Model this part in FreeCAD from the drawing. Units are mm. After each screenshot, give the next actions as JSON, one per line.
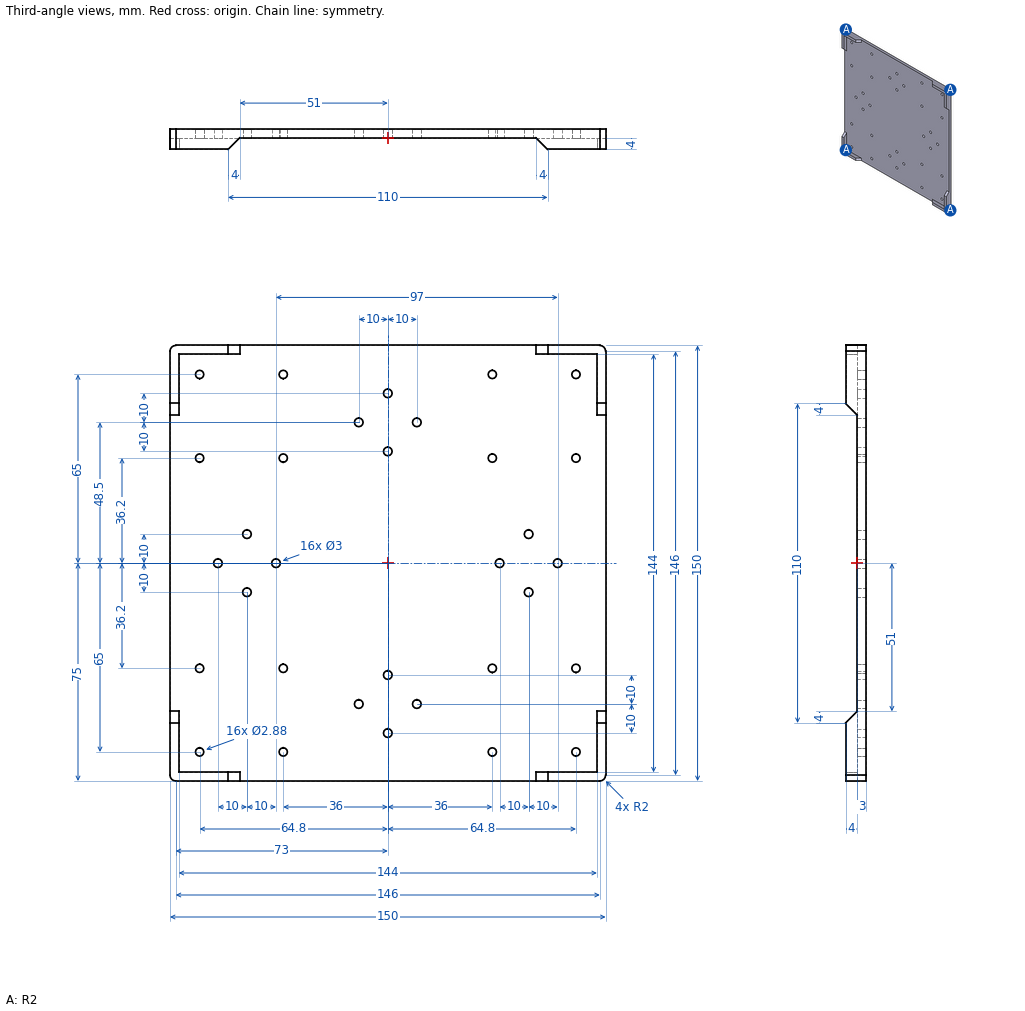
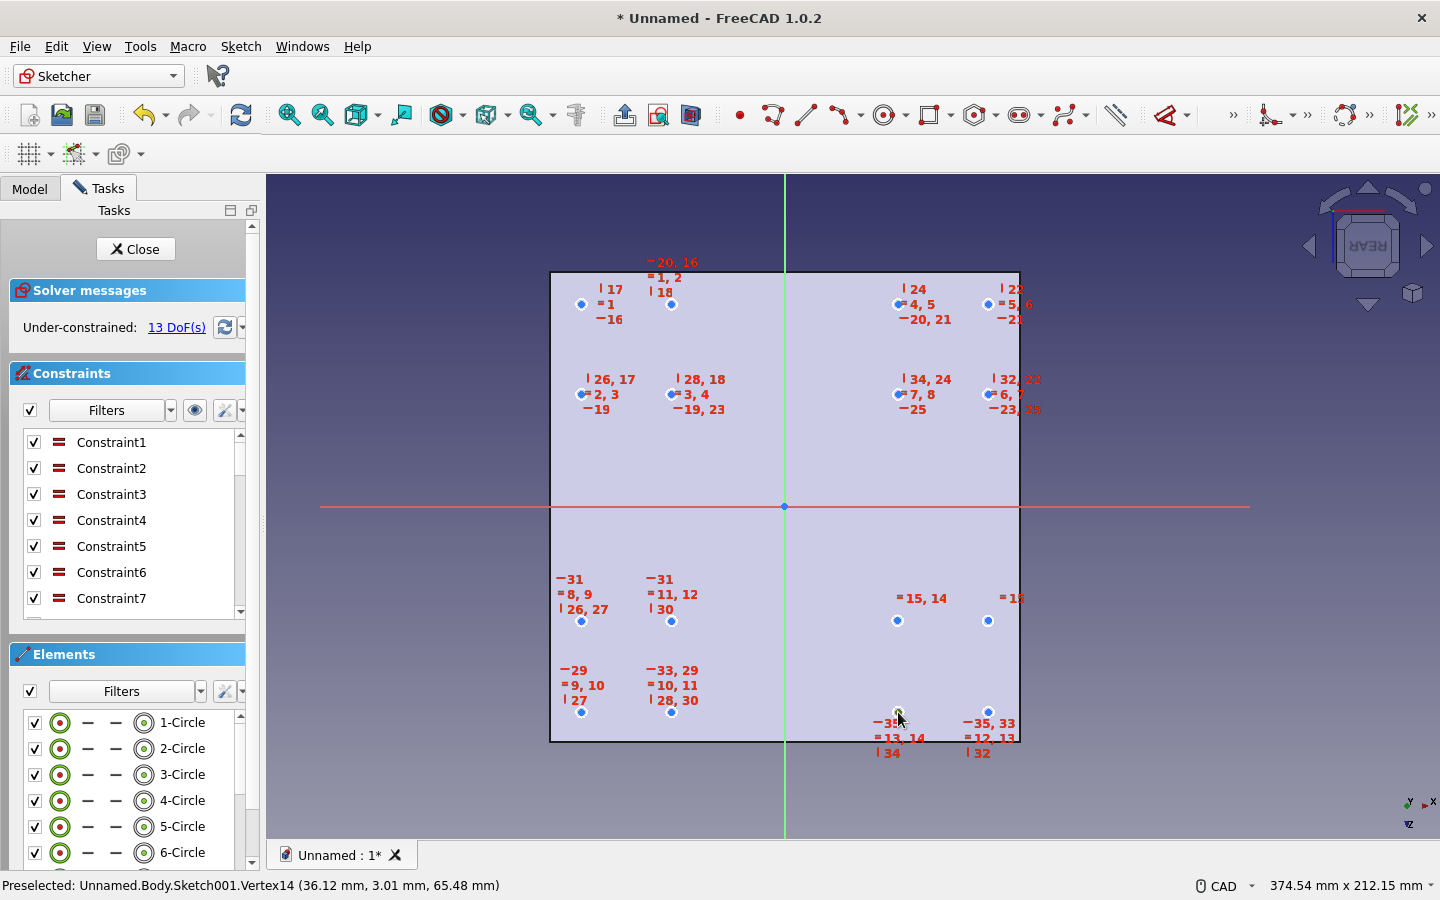
{"action": "left_click", "coordinate": [898, 621]}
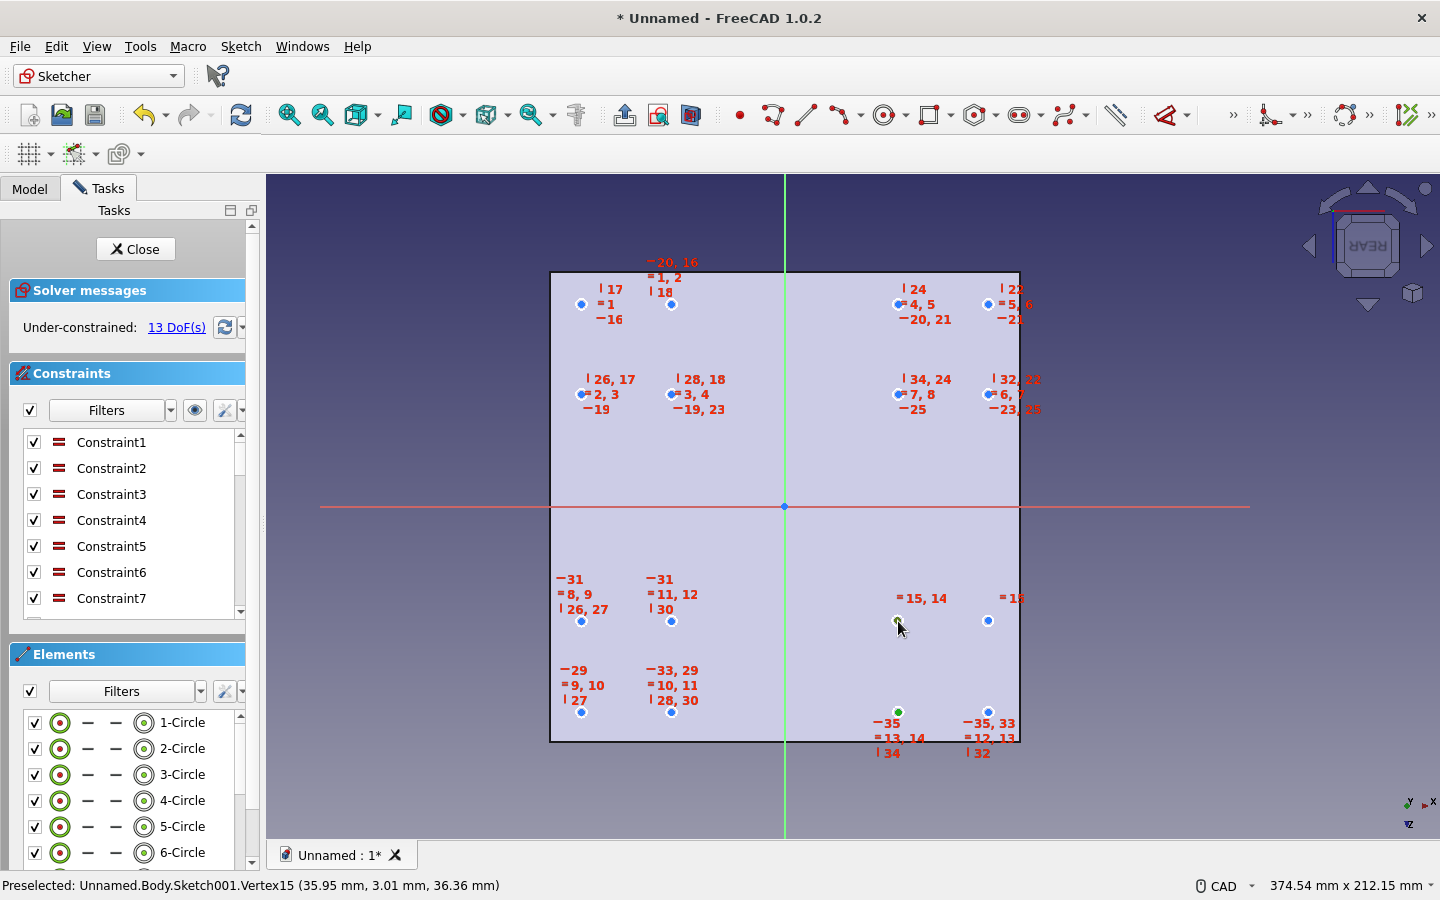
{"action": "key", "text": "v"}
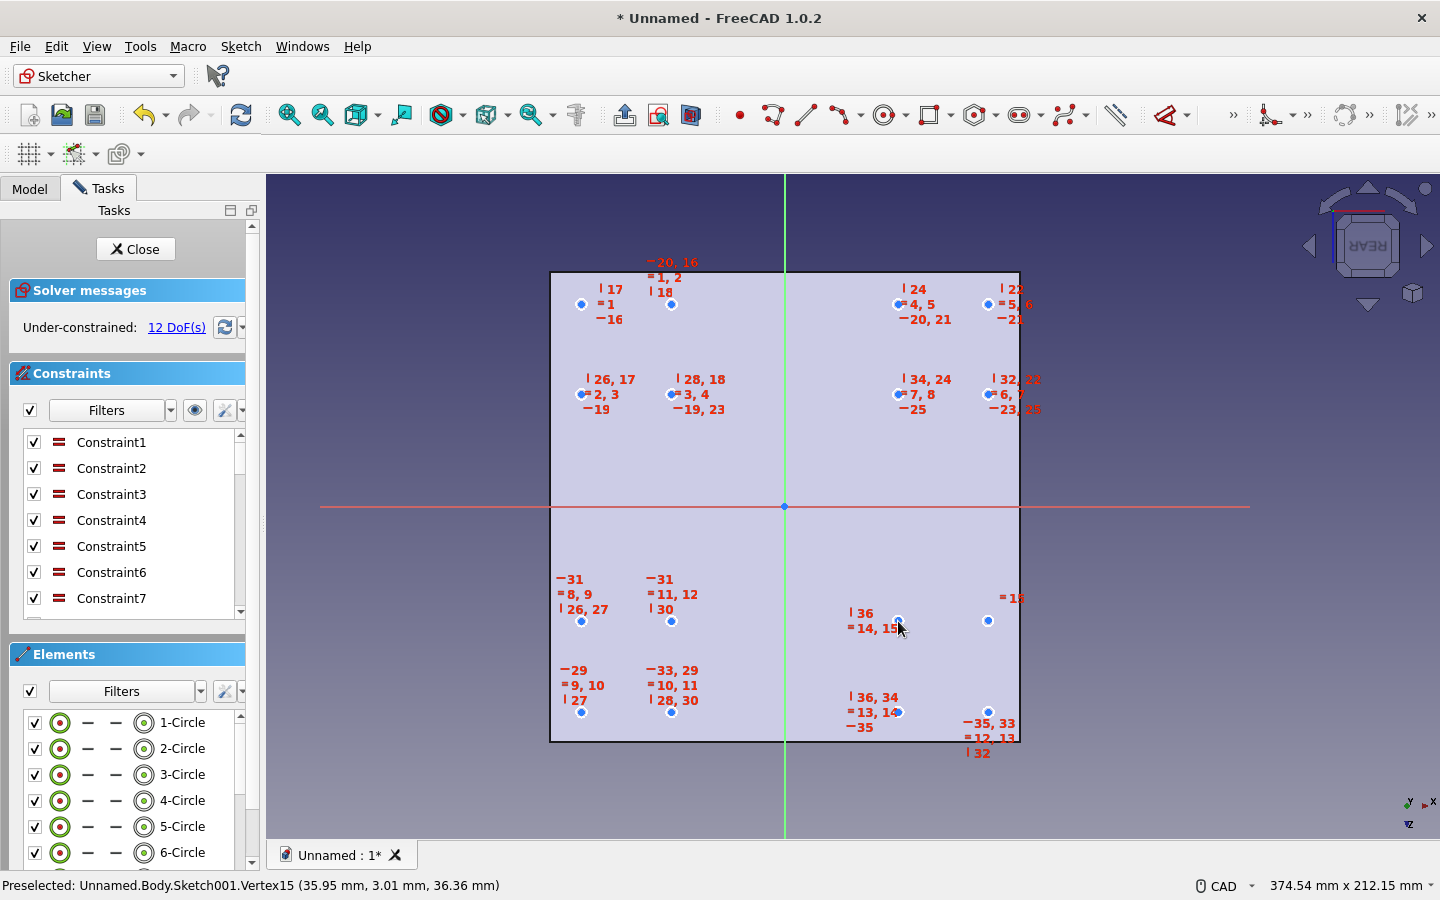
{"action": "left_click", "coordinate": [672, 621]}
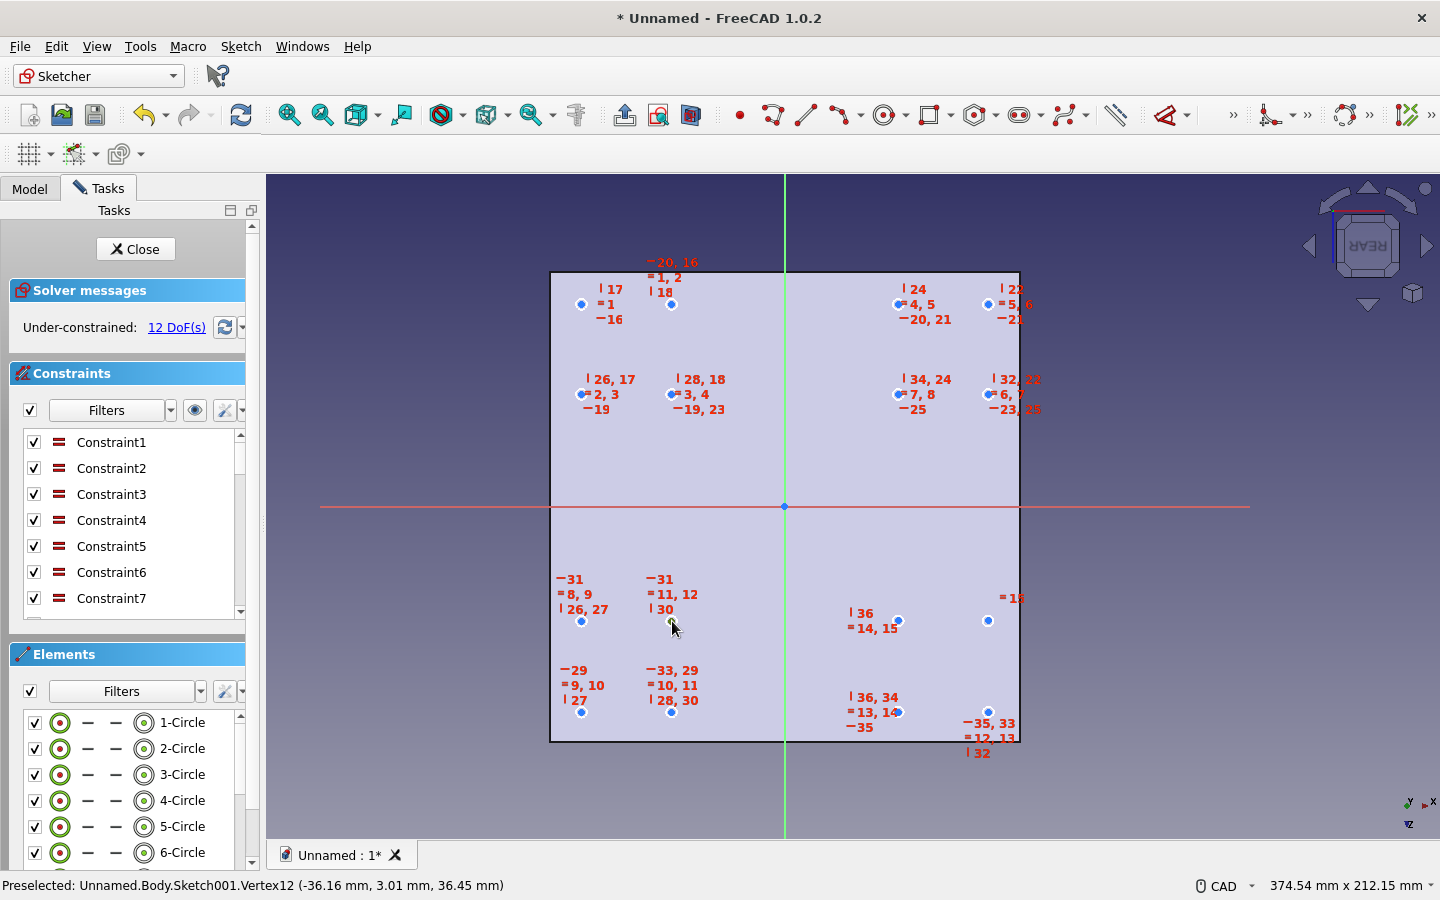
{"action": "left_click", "coordinate": [898, 621]}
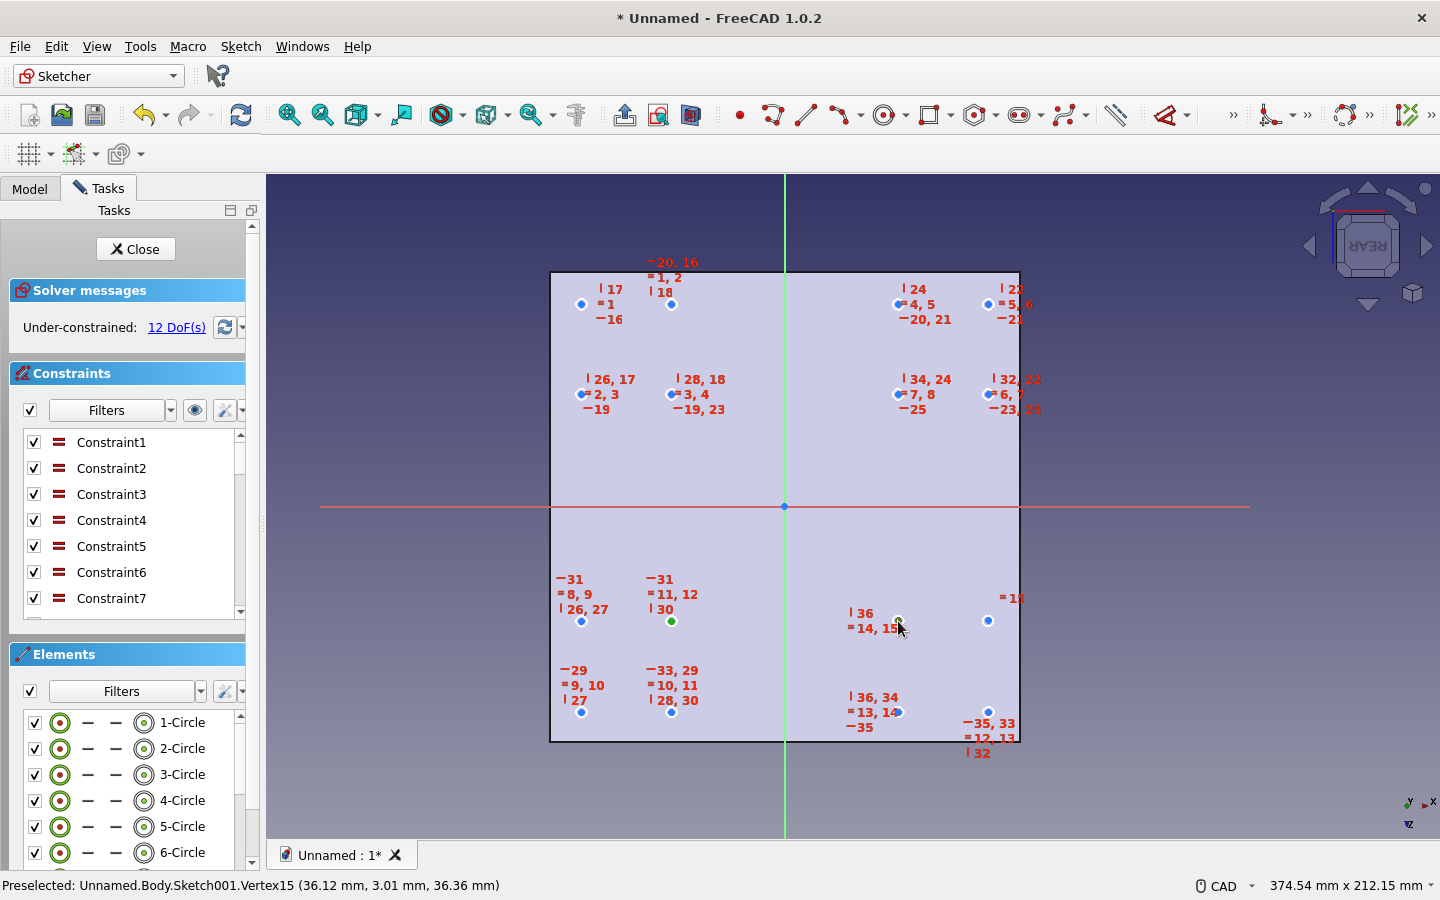
{"action": "key", "text": "h"}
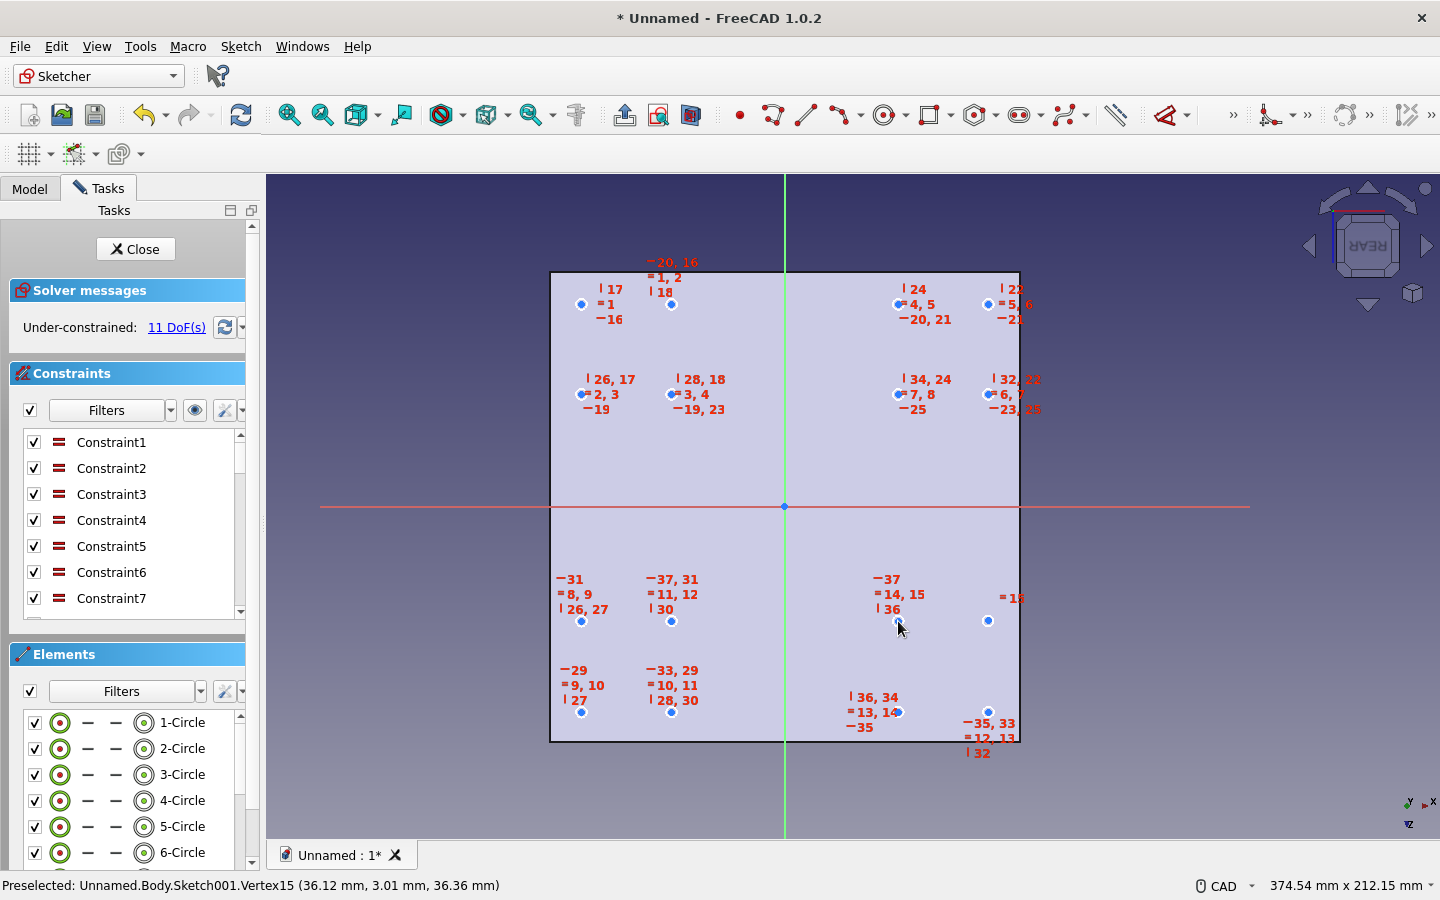
{"action": "left_click", "coordinate": [988, 712]}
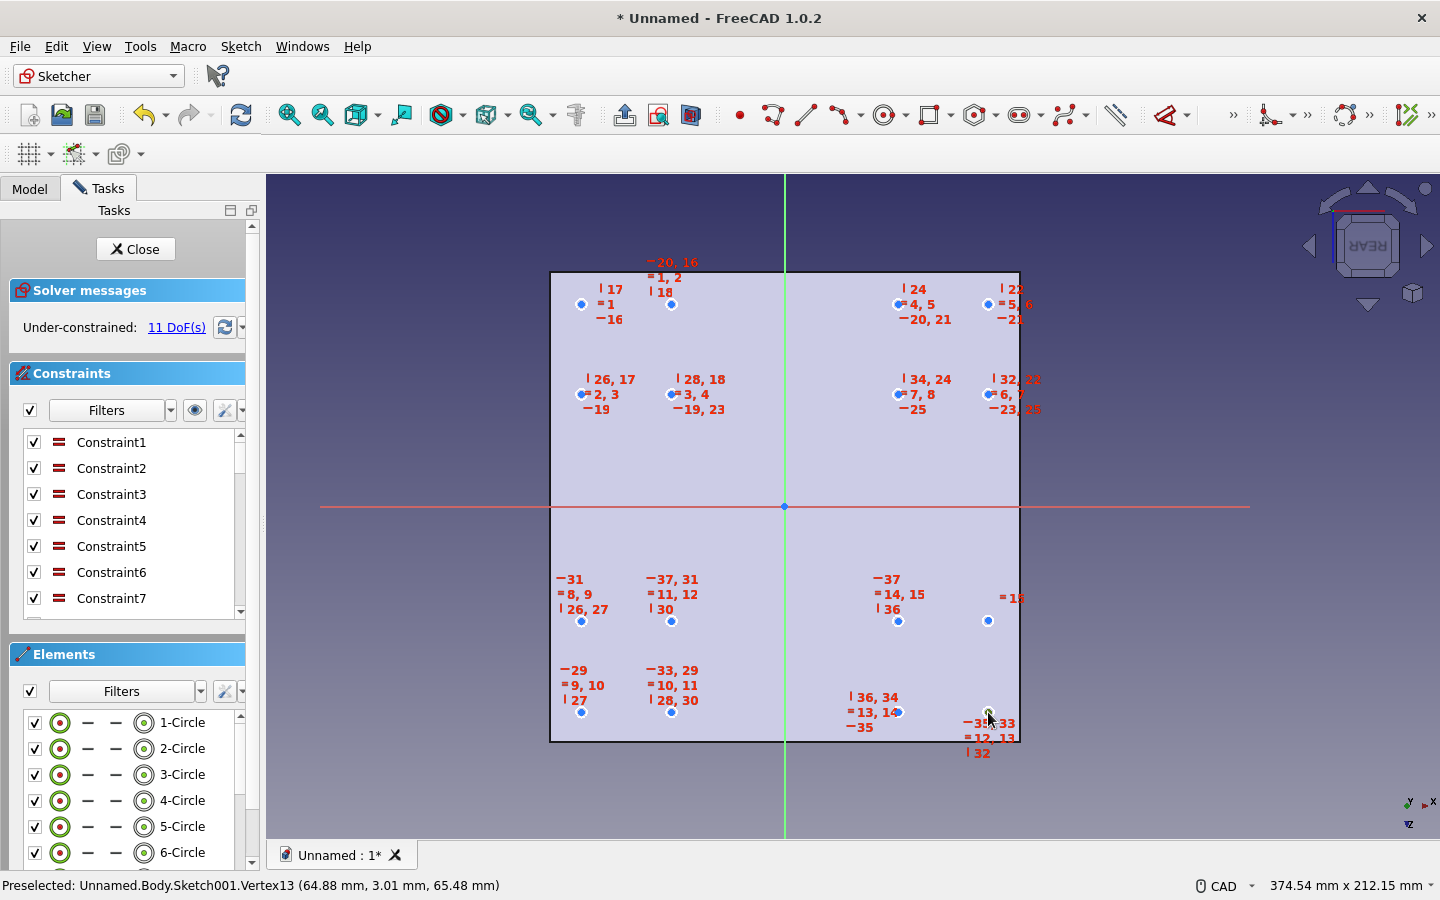
{"action": "left_click", "coordinate": [988, 621]}